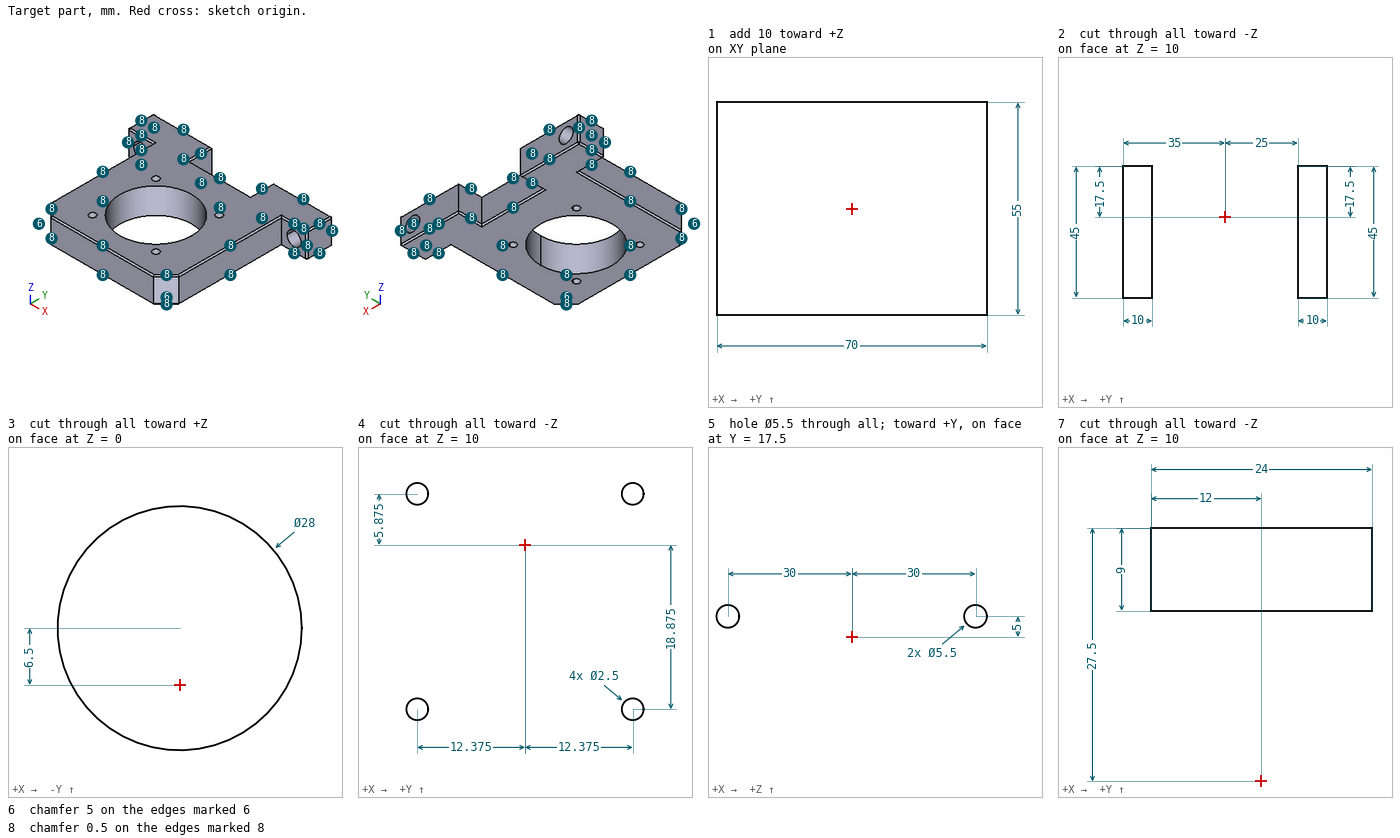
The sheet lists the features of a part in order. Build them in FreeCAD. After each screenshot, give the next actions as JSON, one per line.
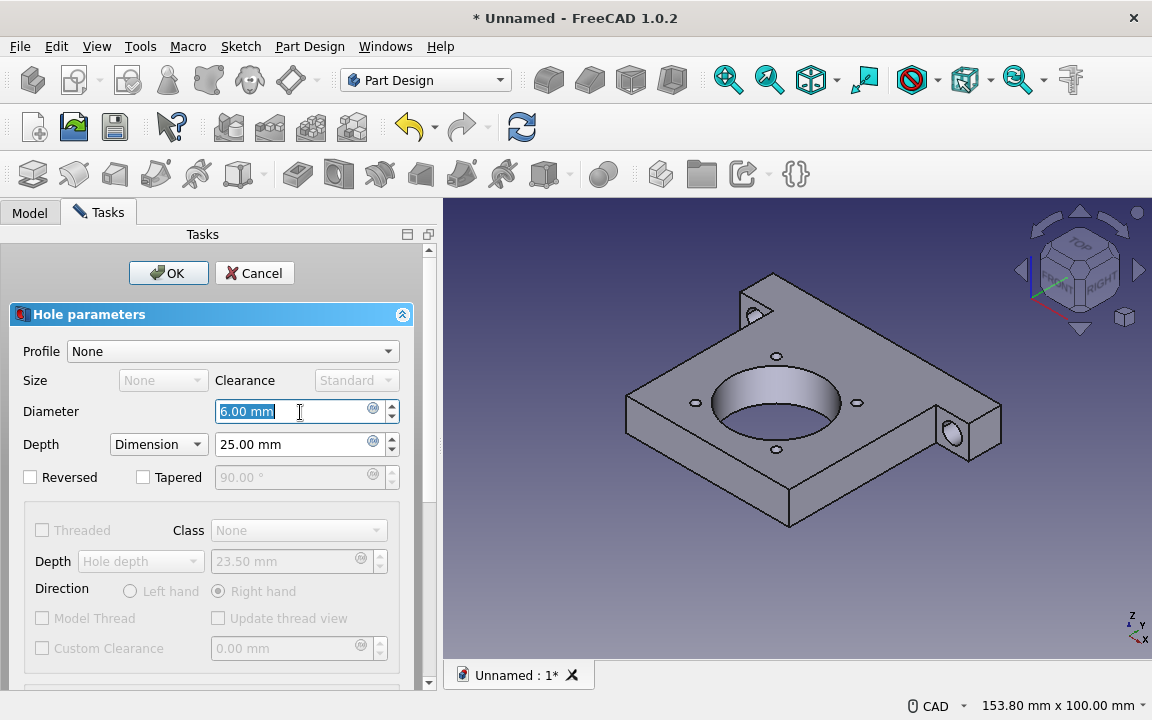
{"action": "type", "text": "5.5"}
{"action": "key", "text": "Tab"}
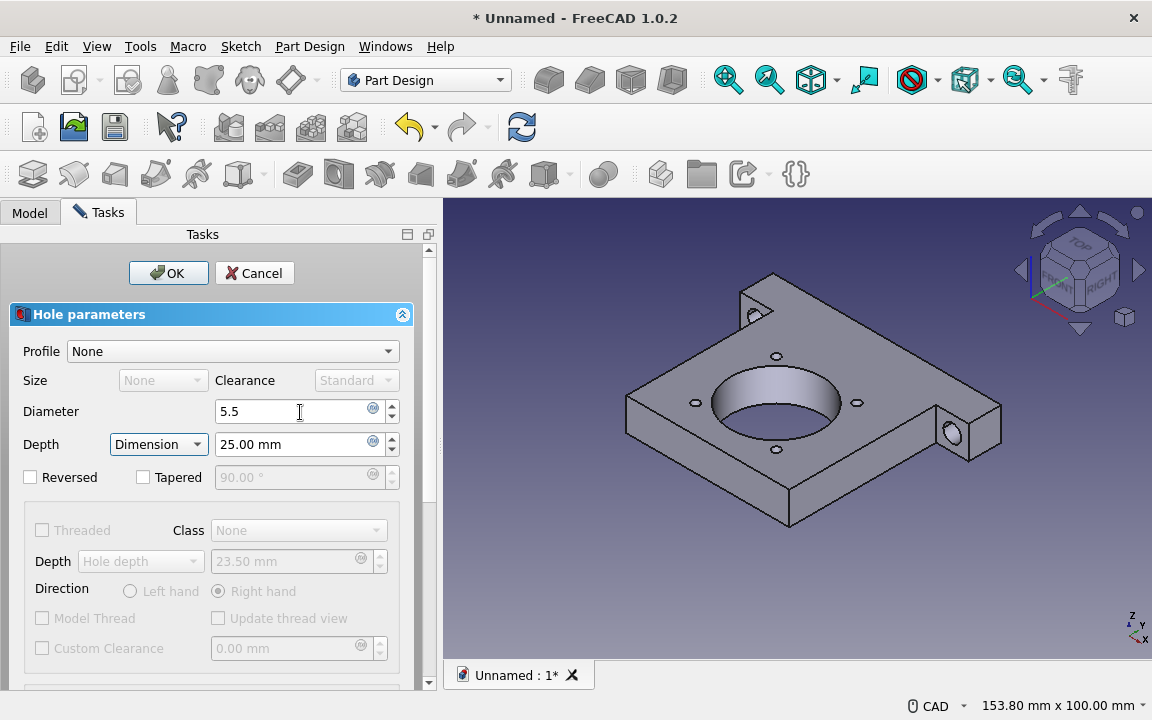
{"action": "left_click", "coordinate": [160, 444]}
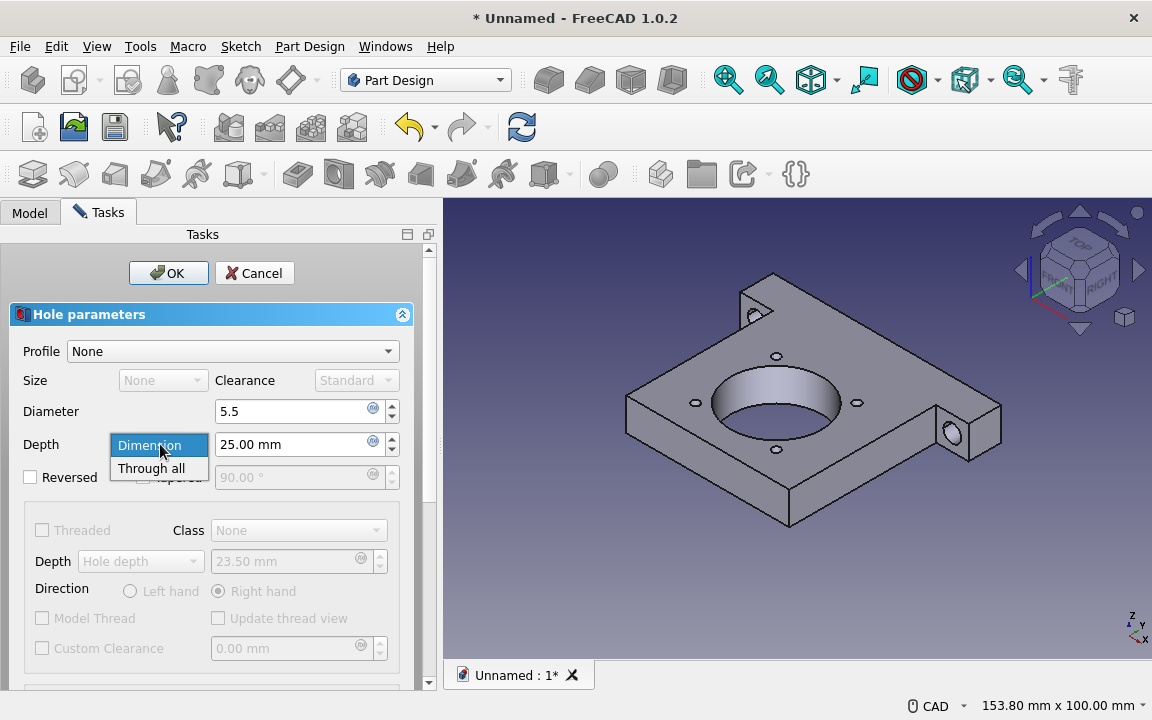
{"action": "left_click", "coordinate": [158, 468]}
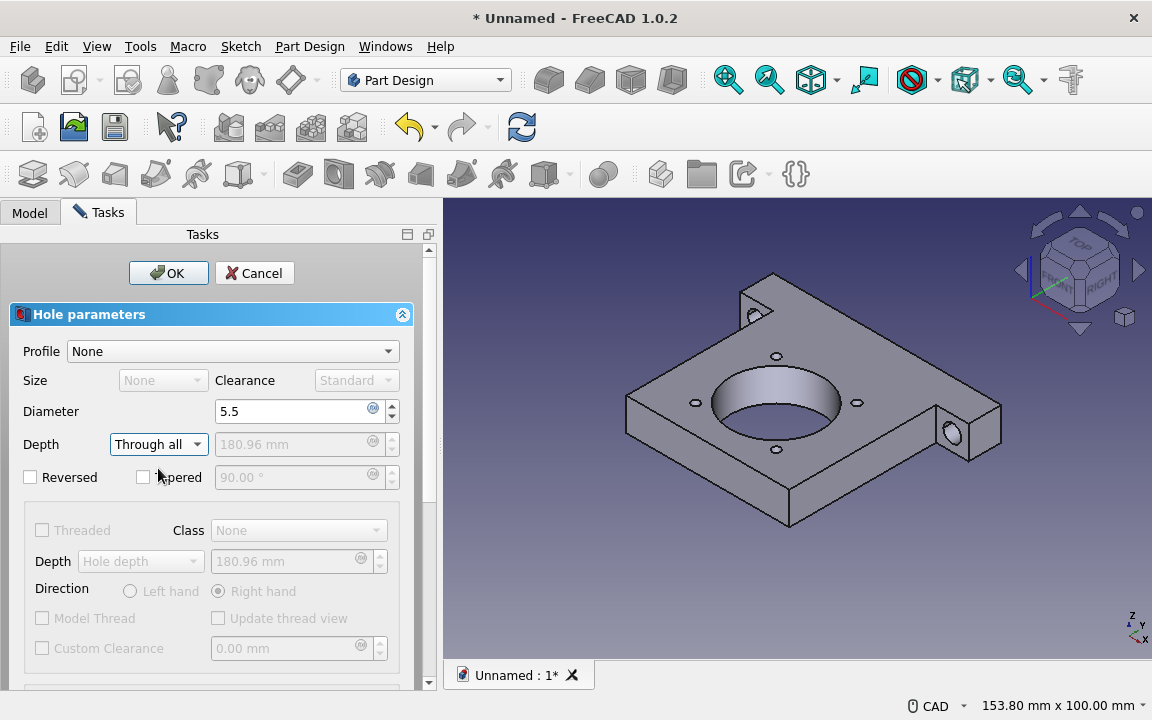
{"action": "left_click", "coordinate": [169, 273]}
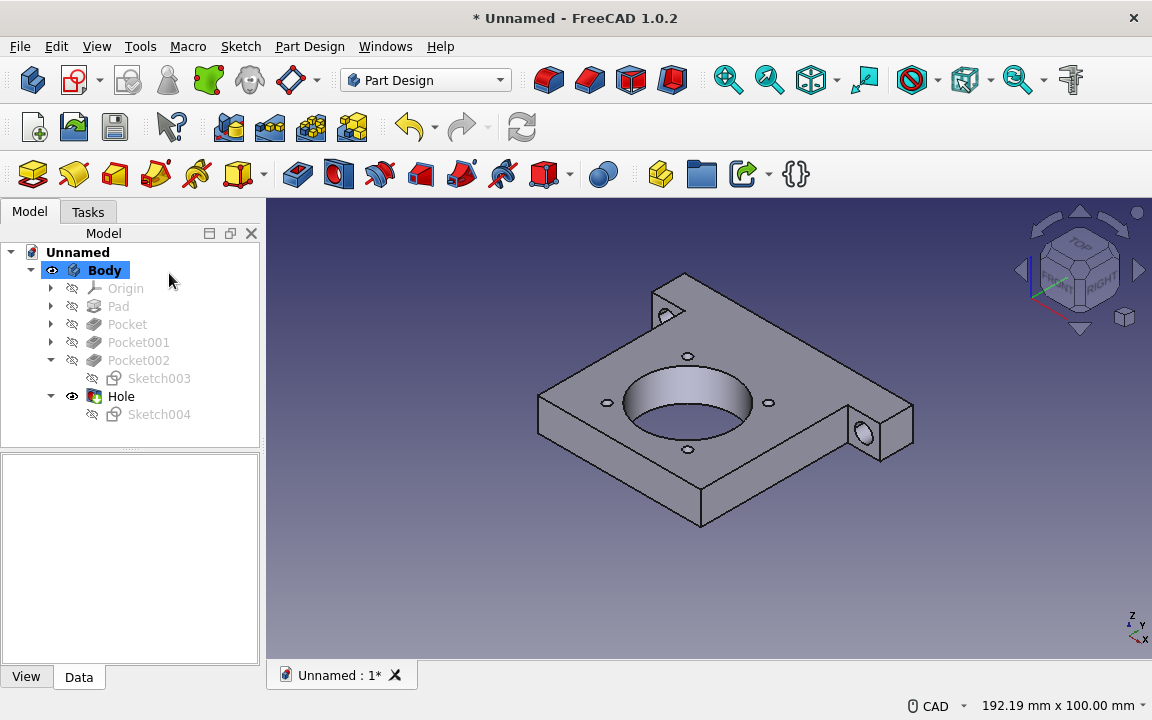
{"action": "left_click", "coordinate": [701, 507]}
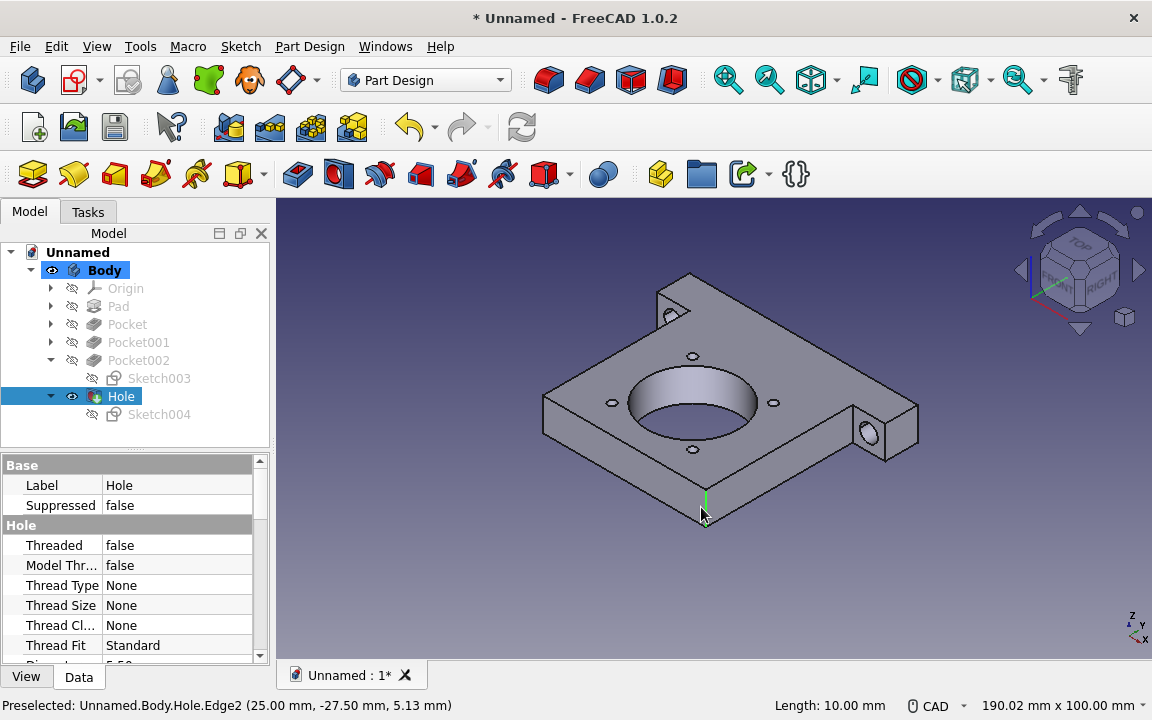
{"action": "key", "text": "2"}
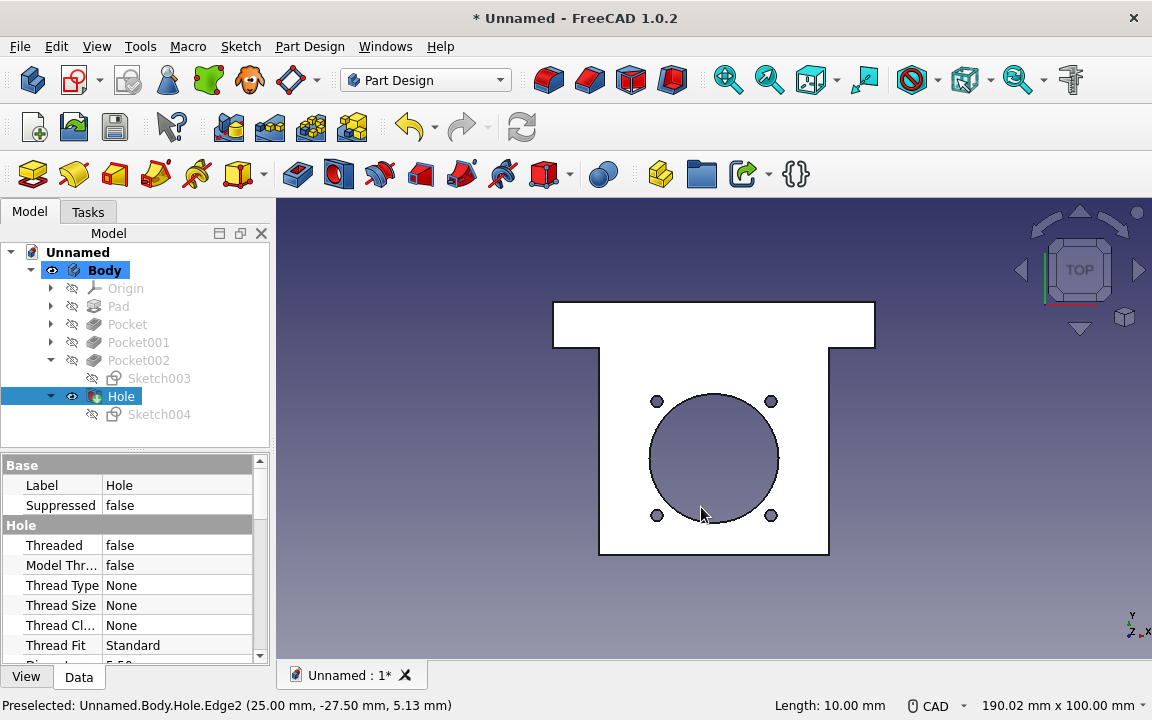
{"action": "key", "text": "0"}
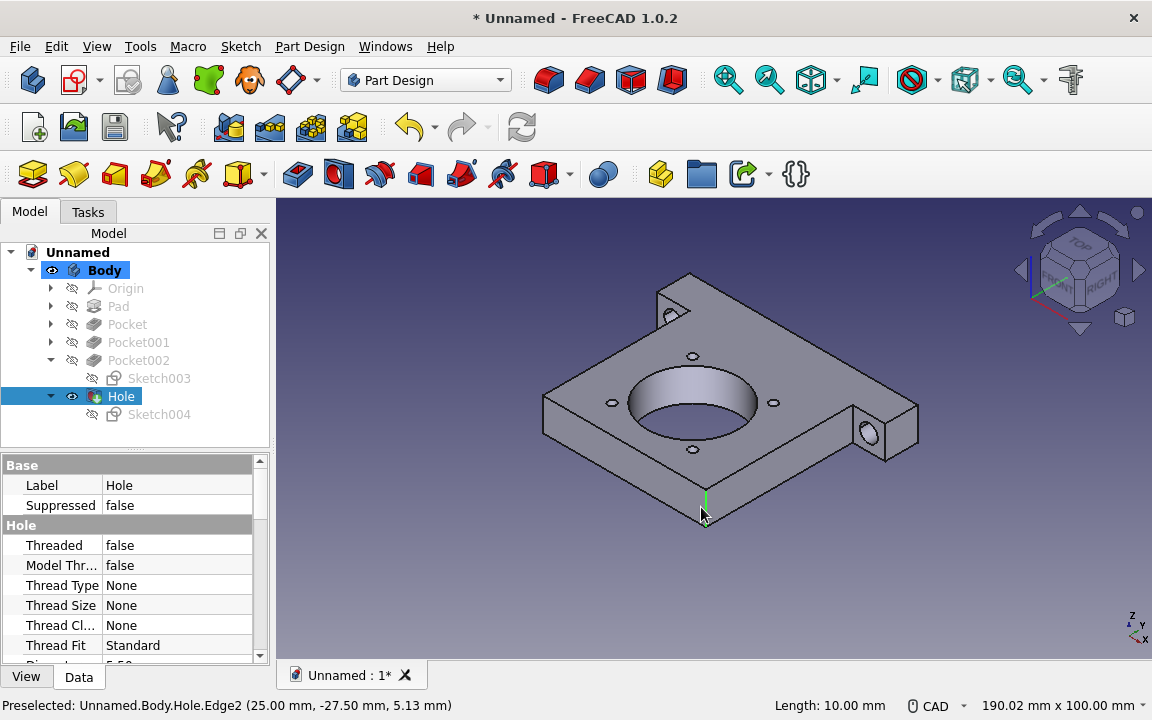
{"action": "key", "text": "1"}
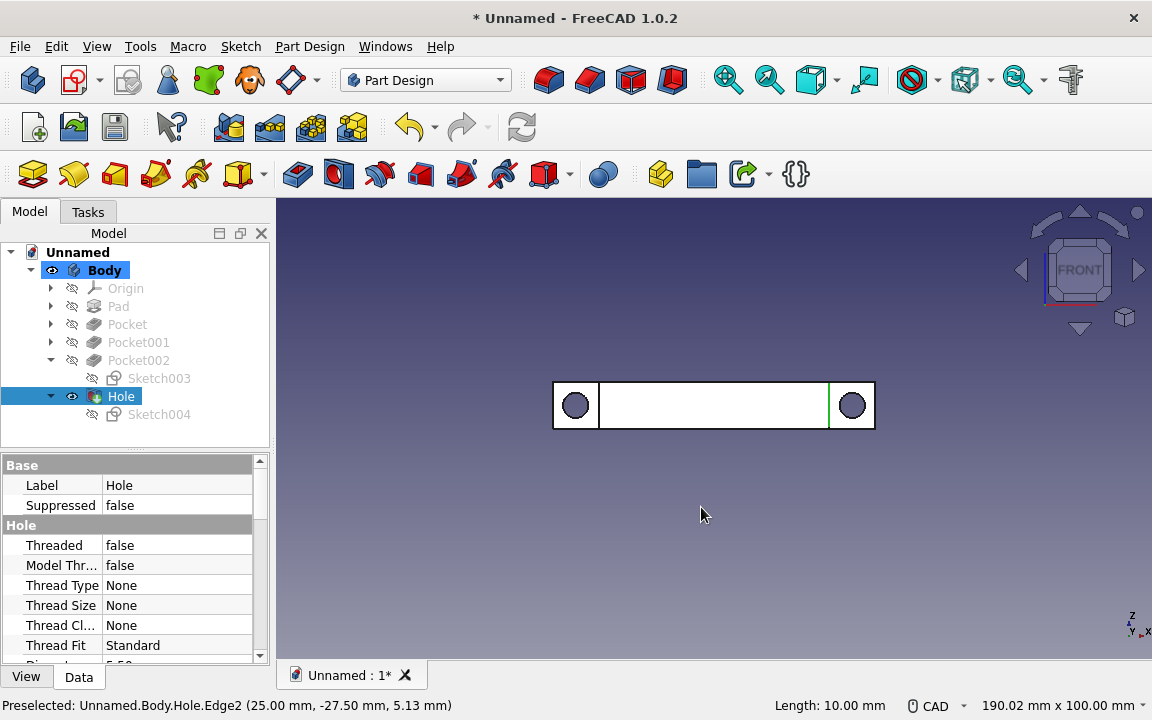
{"action": "left_click", "coordinate": [729, 80]}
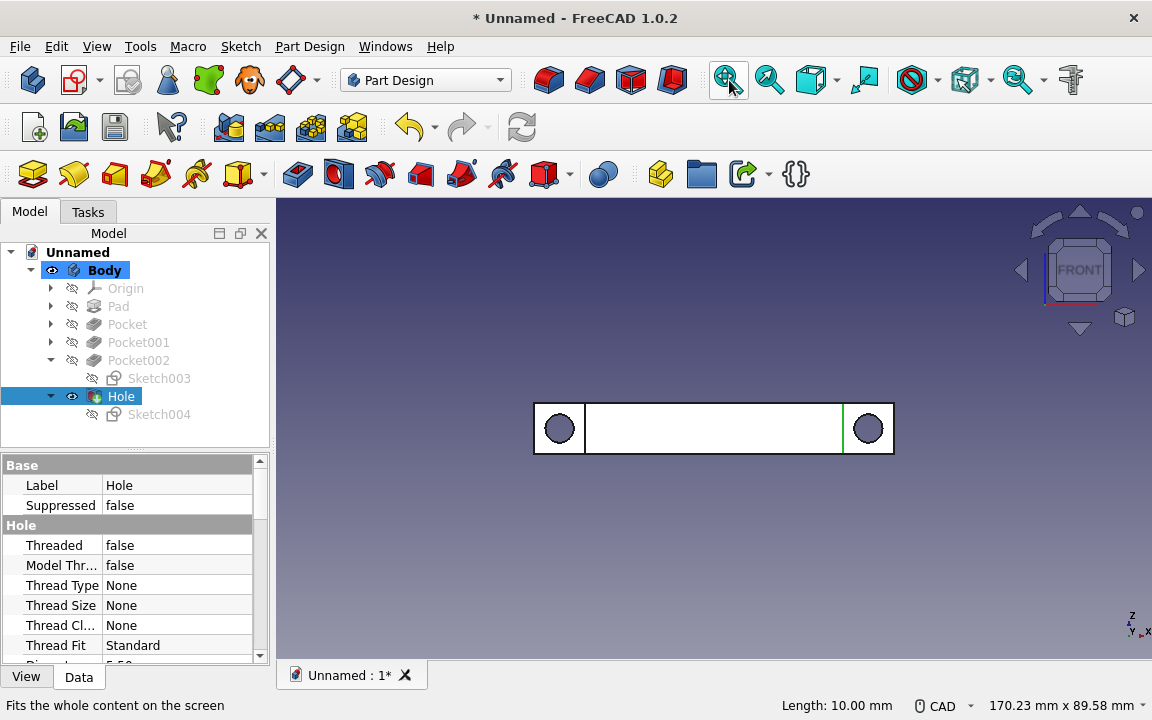
{"action": "left_click", "coordinate": [585, 428], "text": "ctrl"}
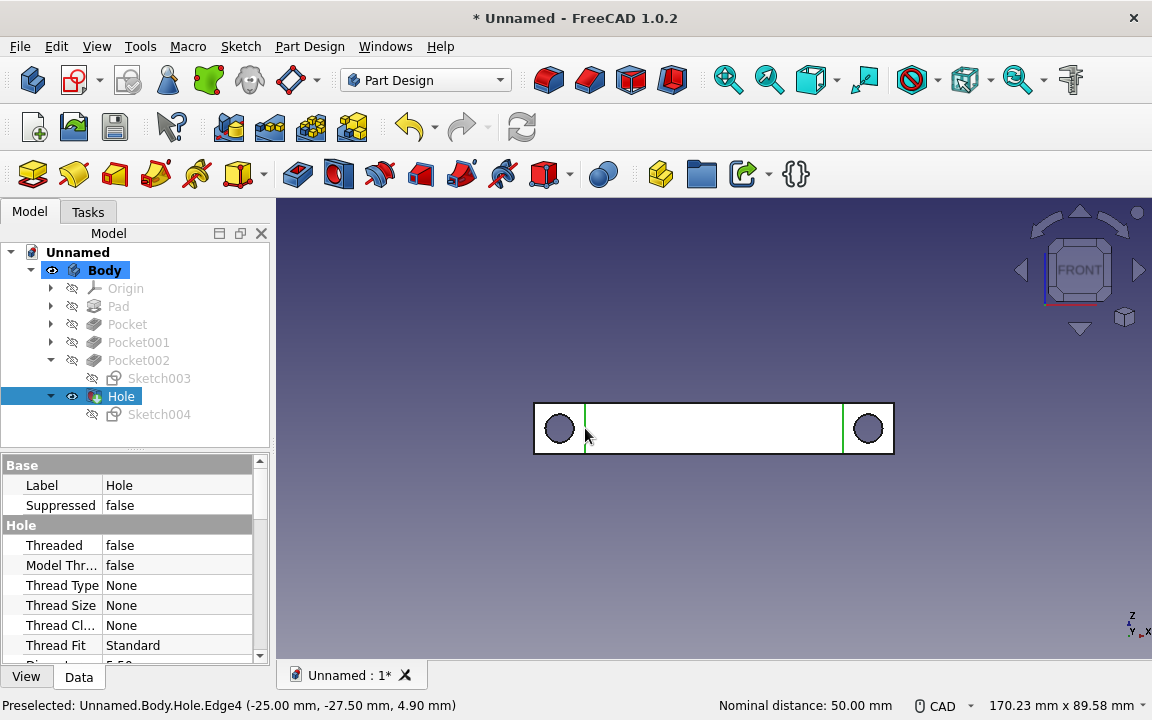
{"action": "left_click", "coordinate": [590, 80]}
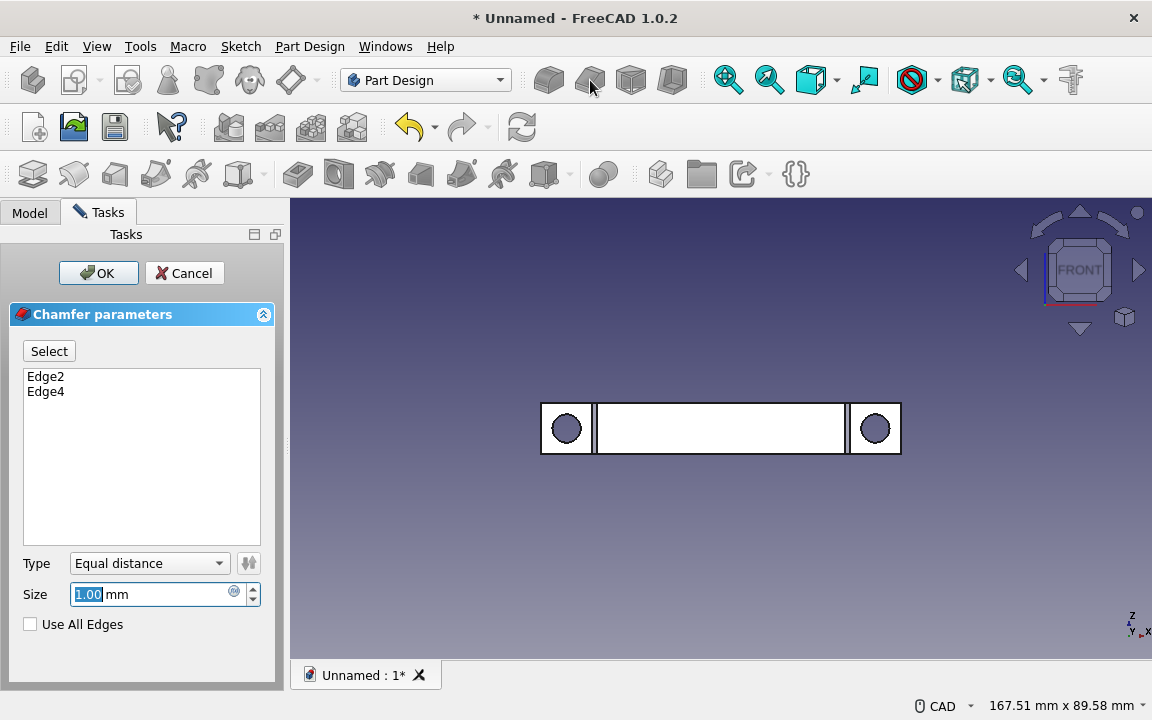
{"action": "type", "text": "5"}
{"action": "key", "text": "Tab"}